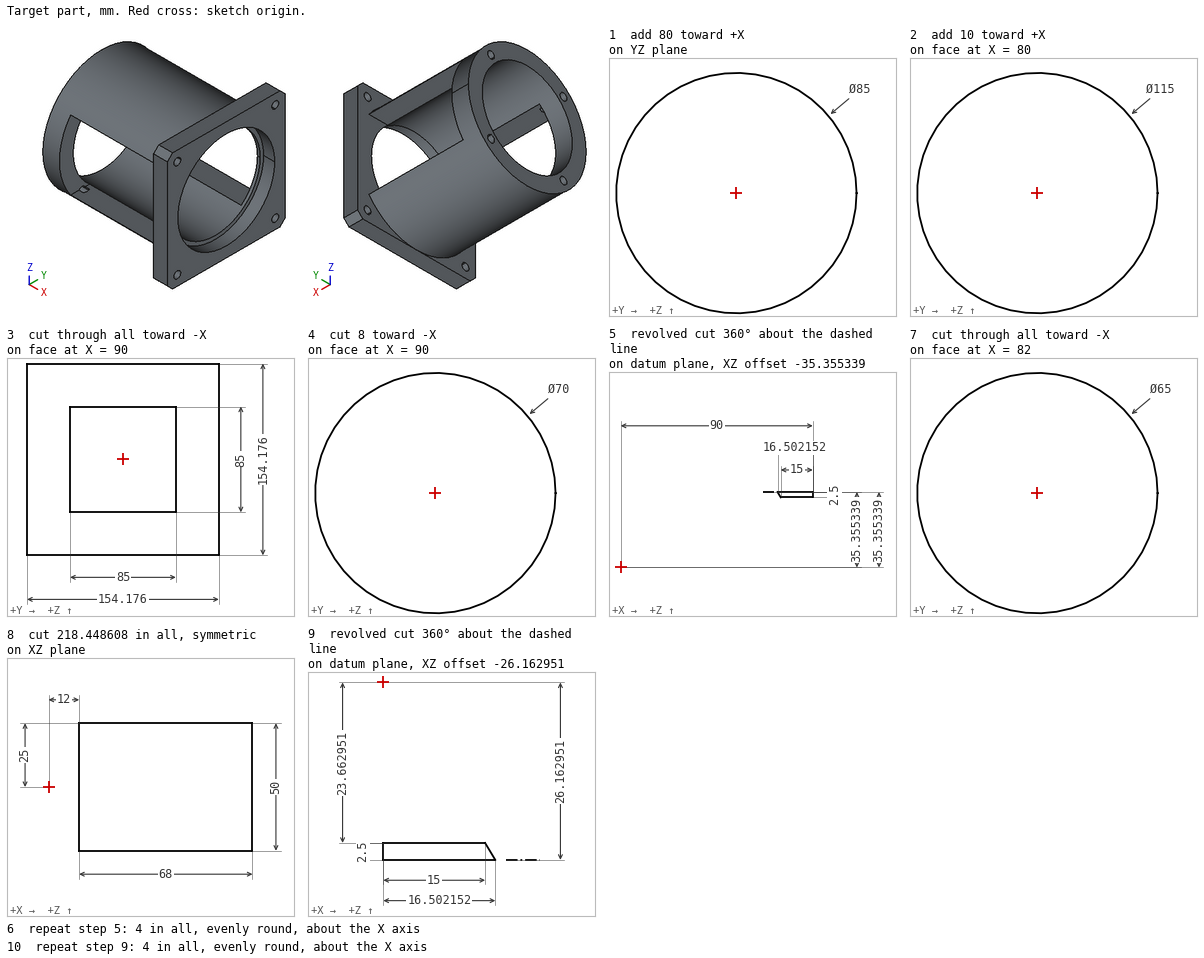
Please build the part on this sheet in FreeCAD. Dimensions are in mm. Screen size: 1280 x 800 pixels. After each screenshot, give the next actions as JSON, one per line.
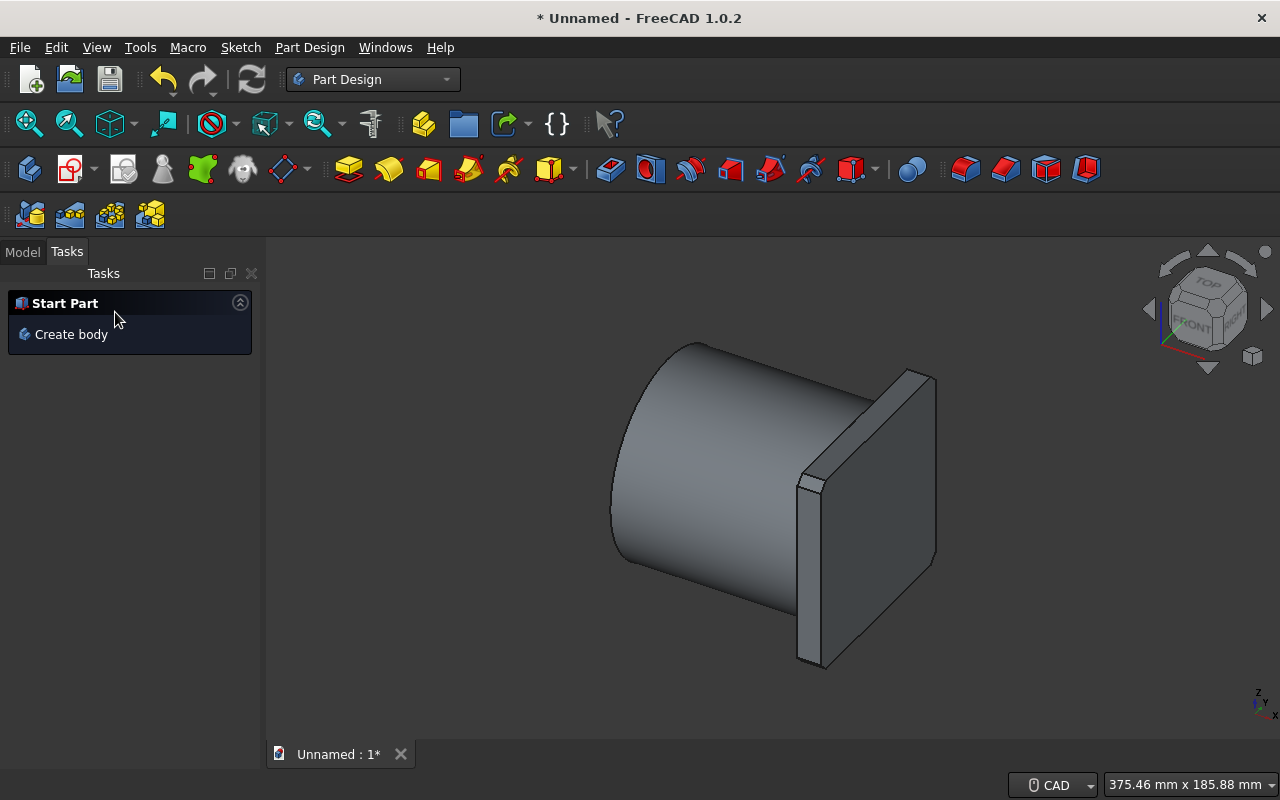
{"action": "left_click", "coordinate": [878, 522]}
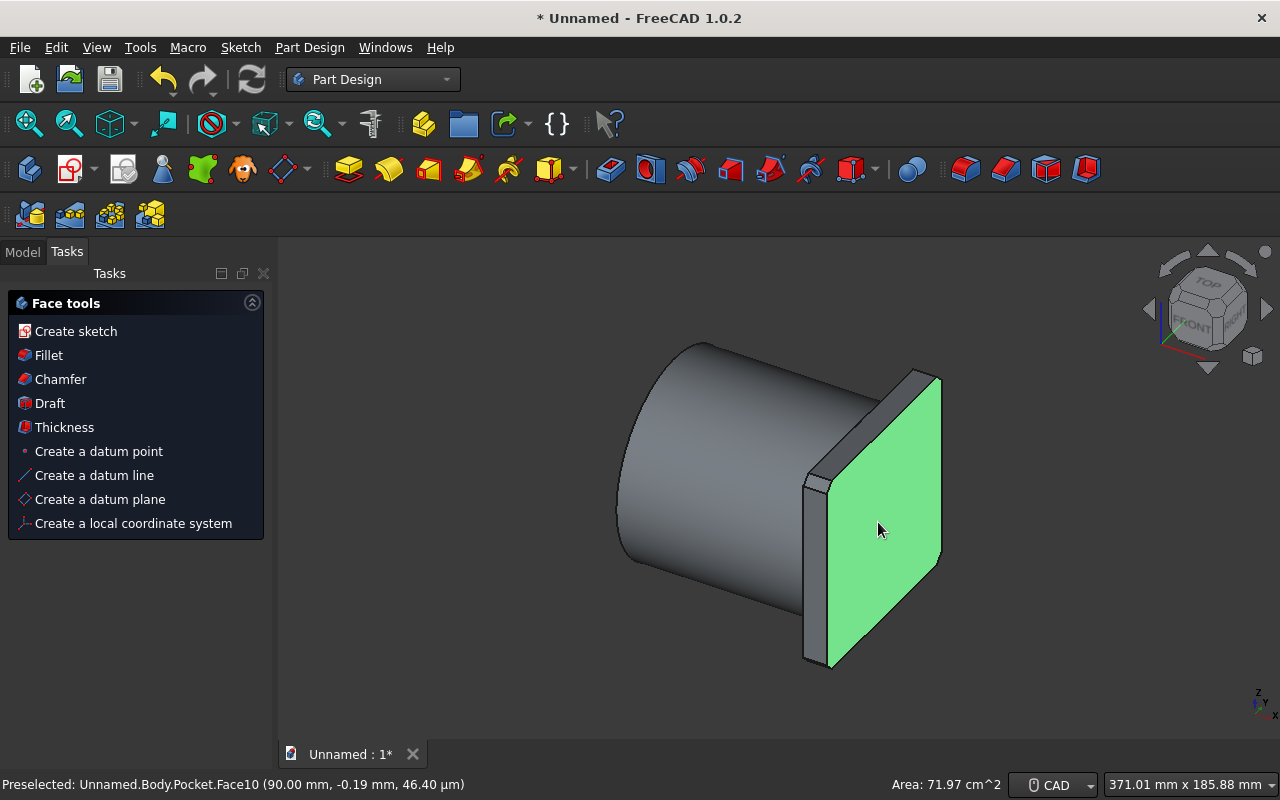
{"action": "left_click", "coordinate": [70, 170]}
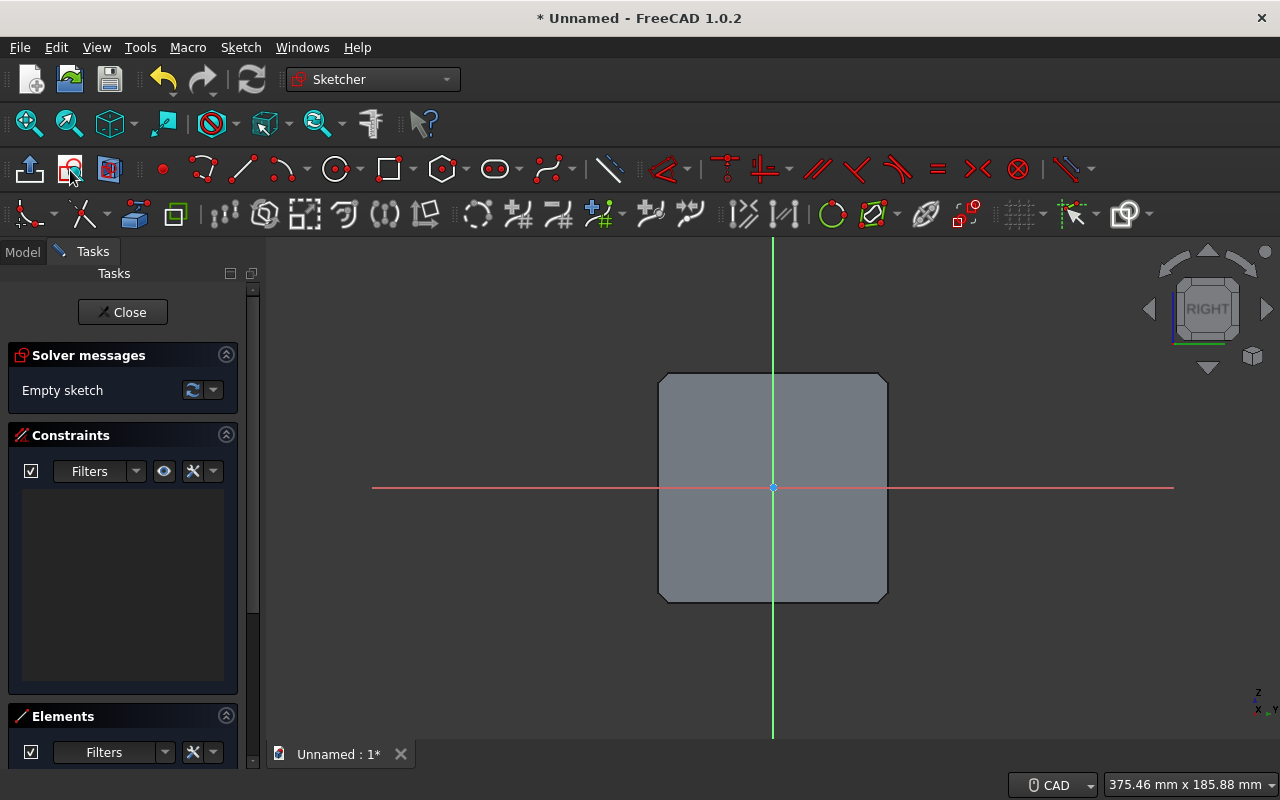
{"action": "scroll", "coordinate": [856, 488], "scroll_direction": "up", "scroll_amount": 3}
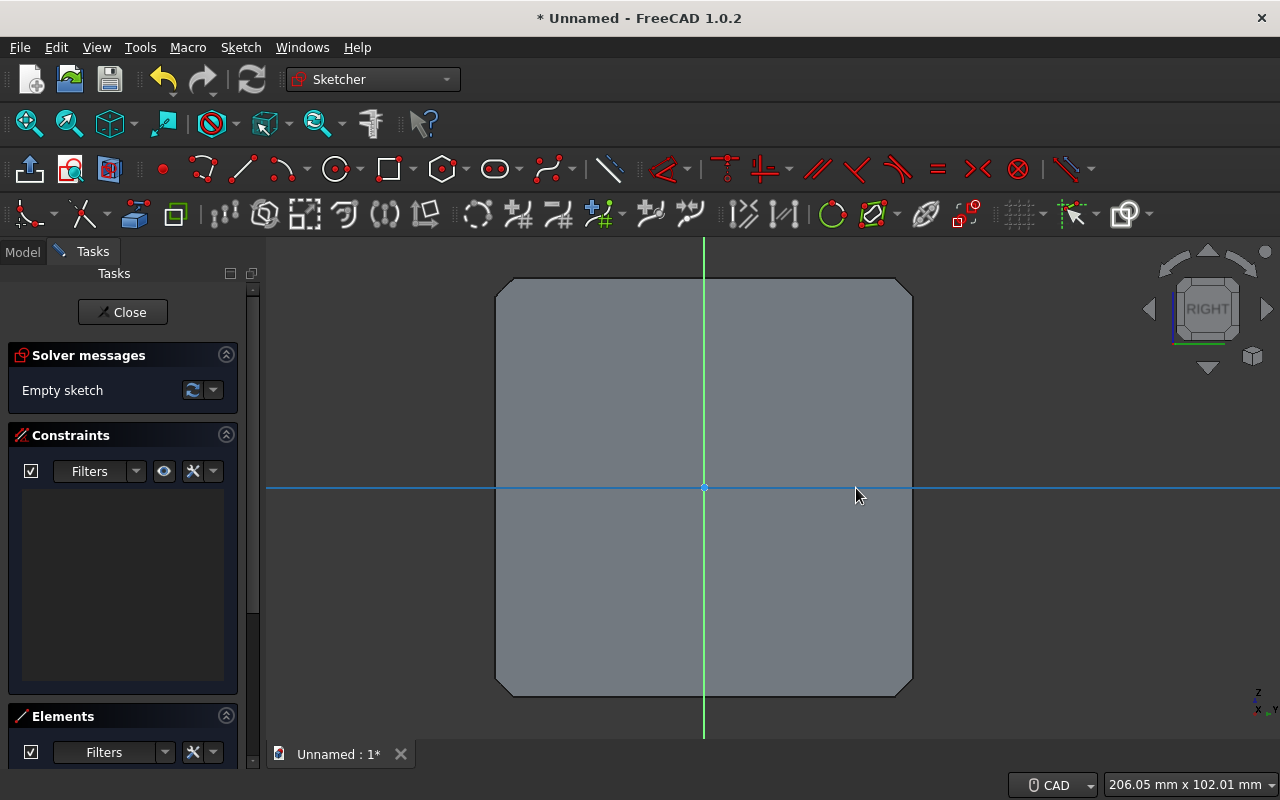
{"action": "left_click", "coordinate": [336, 170]}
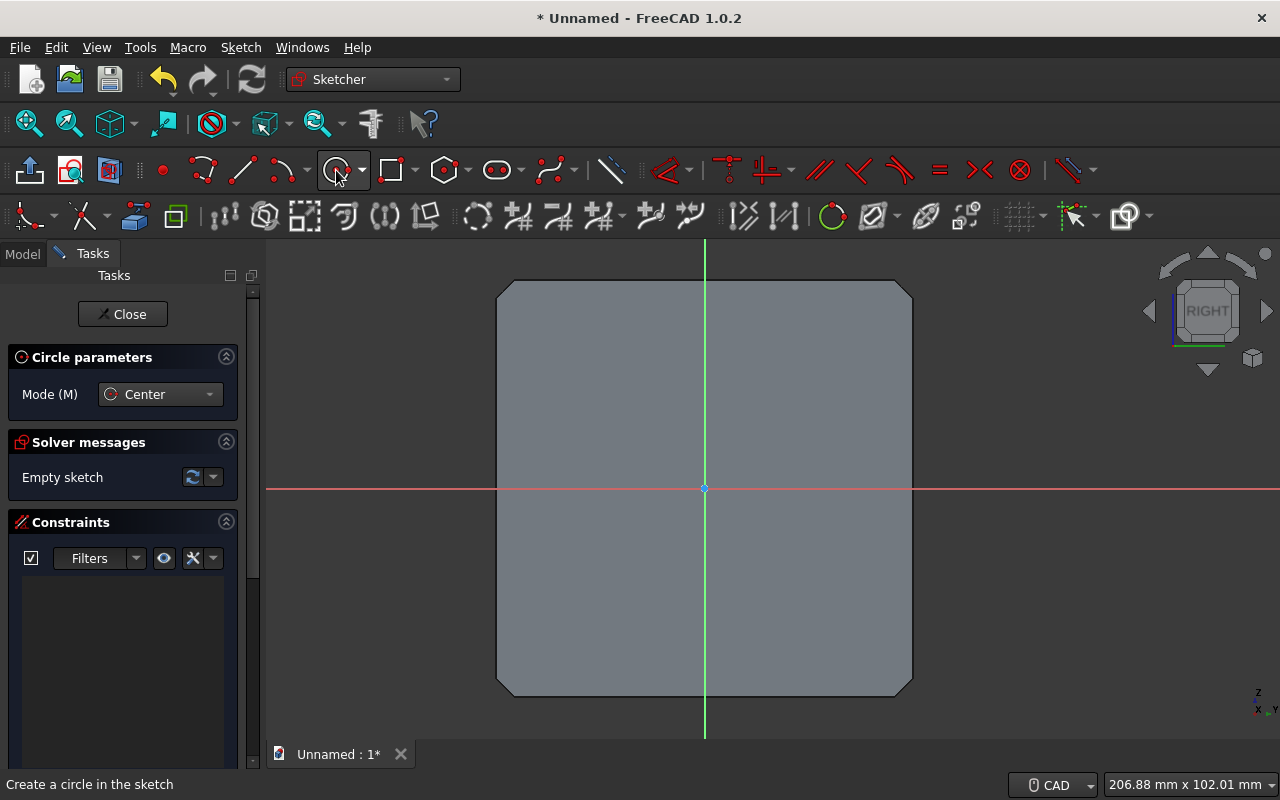
{"action": "left_click", "coordinate": [705, 489]}
{"action": "mouse_move", "coordinate": [826, 367]}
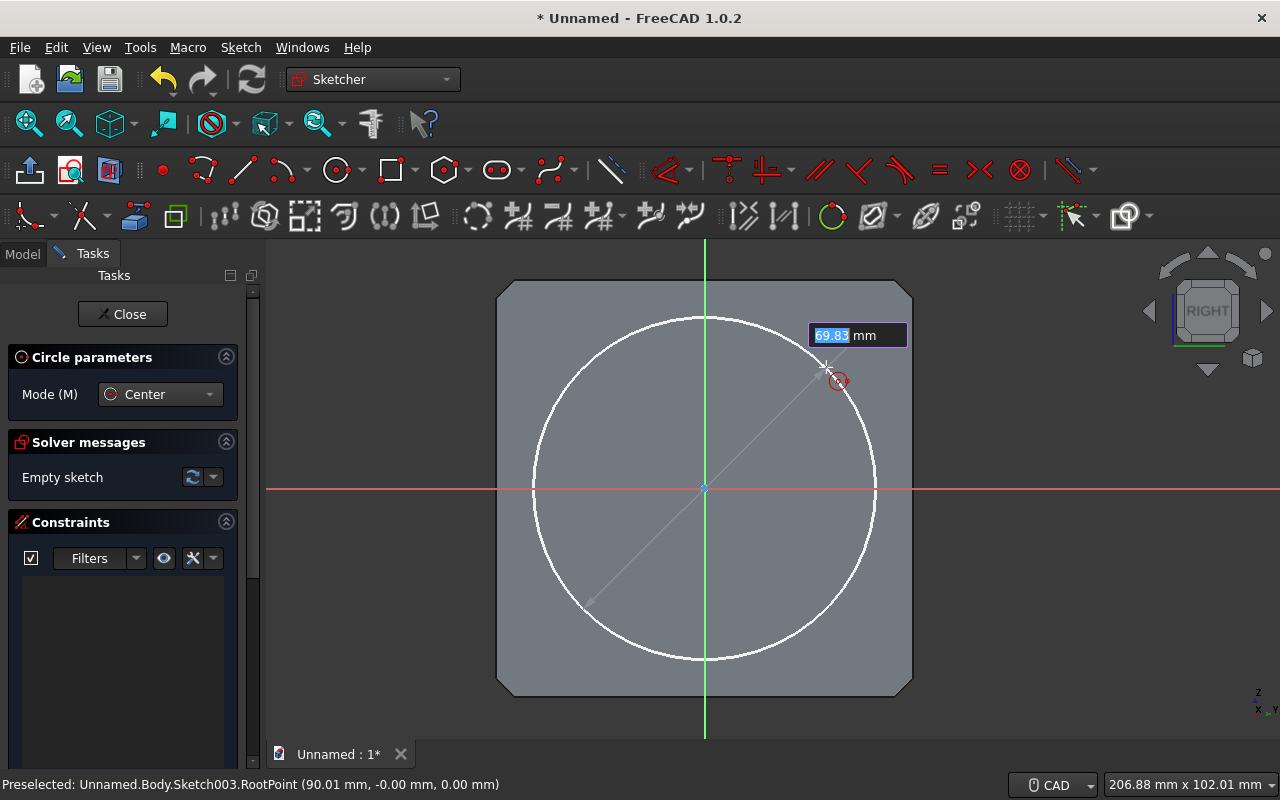
{"action": "type", "text": "70"}
{"action": "key", "text": "Return"}
{"action": "key", "text": "Escape"}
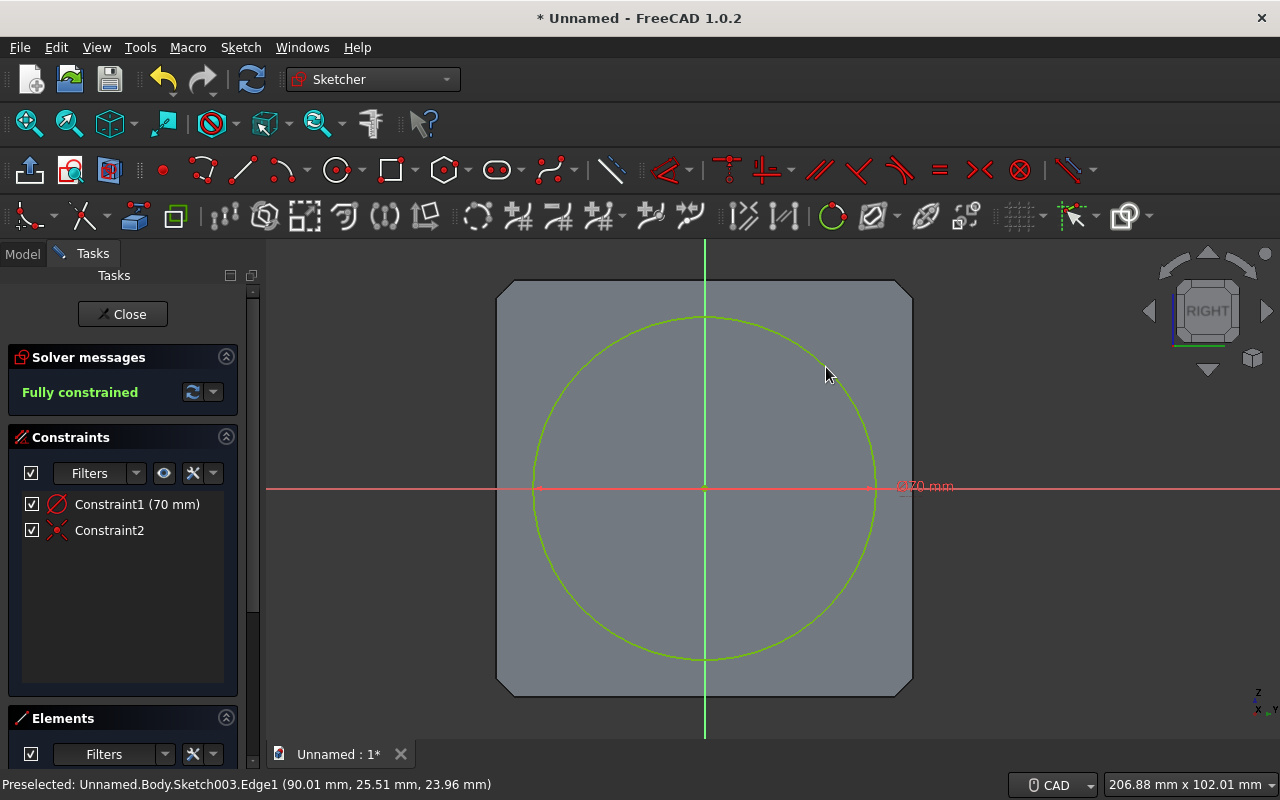
{"action": "left_click", "coordinate": [123, 314]}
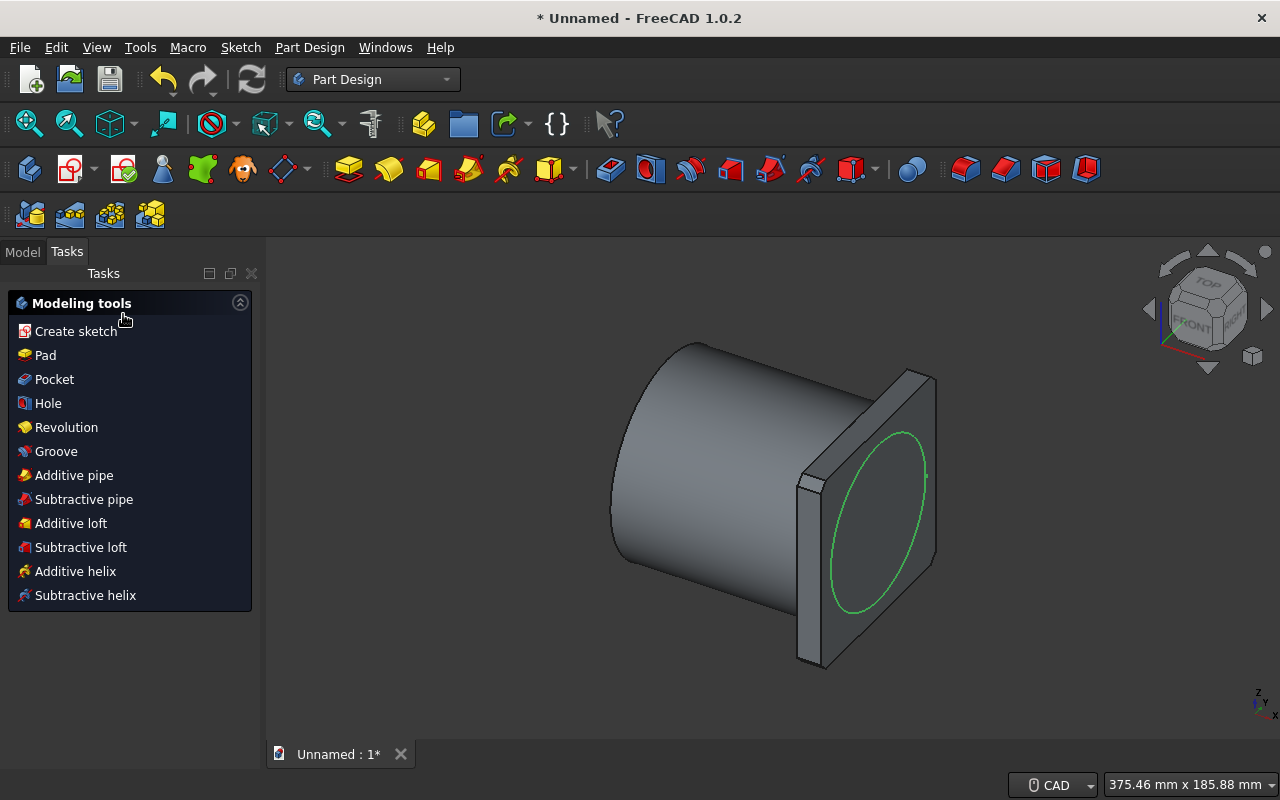
{"action": "left_click", "coordinate": [612, 170]}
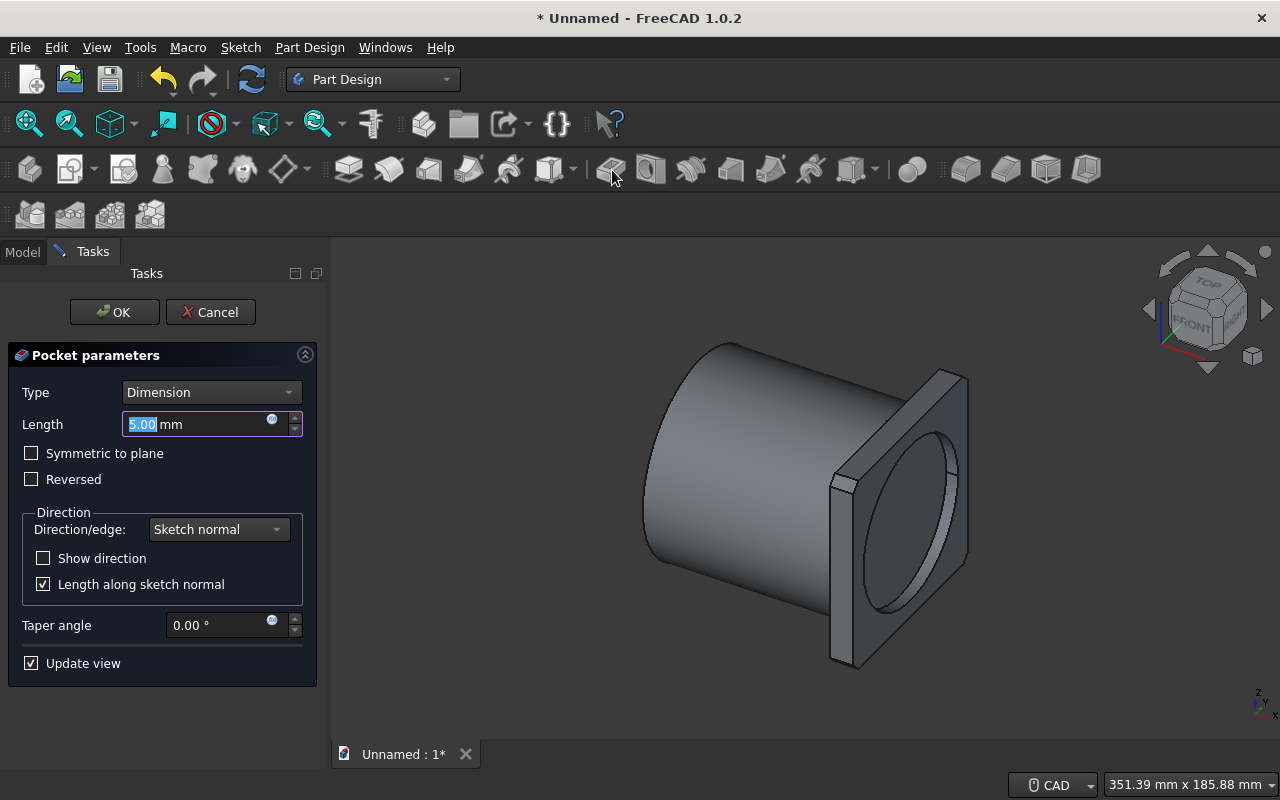
{"action": "type", "text": "8"}
{"action": "key", "text": "Tab"}